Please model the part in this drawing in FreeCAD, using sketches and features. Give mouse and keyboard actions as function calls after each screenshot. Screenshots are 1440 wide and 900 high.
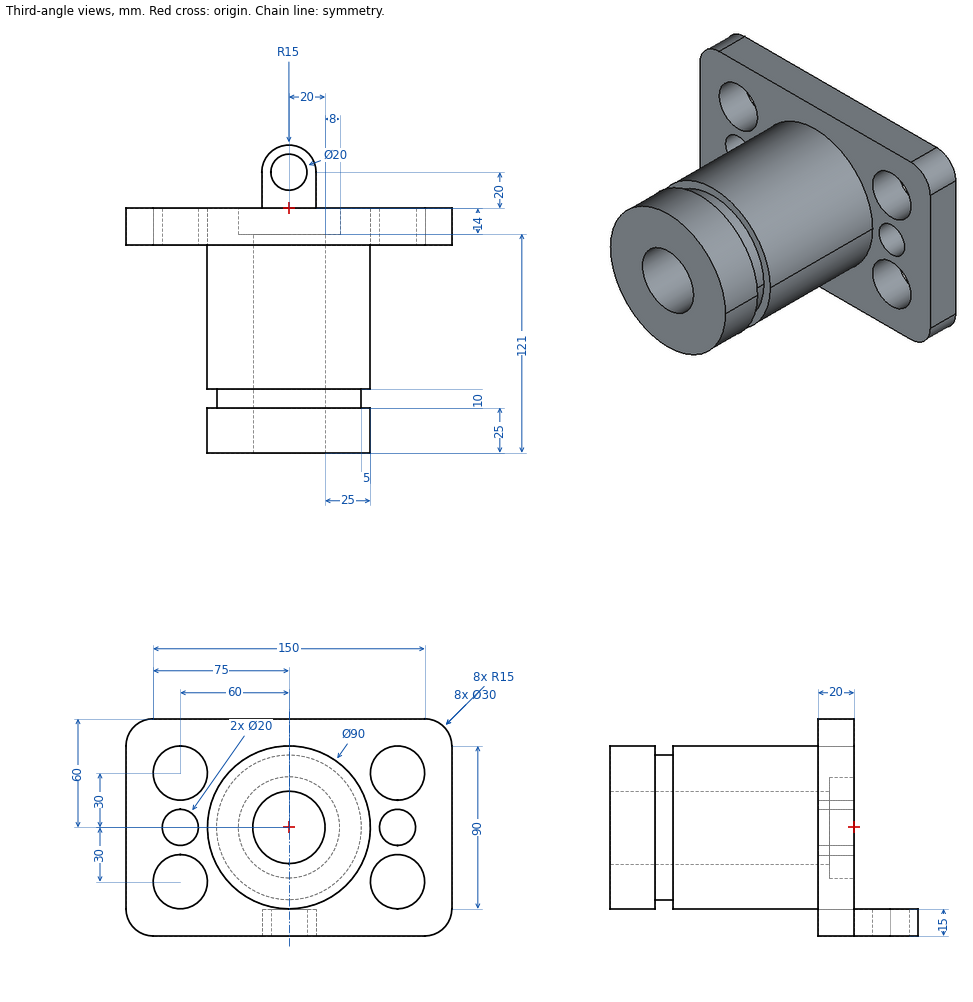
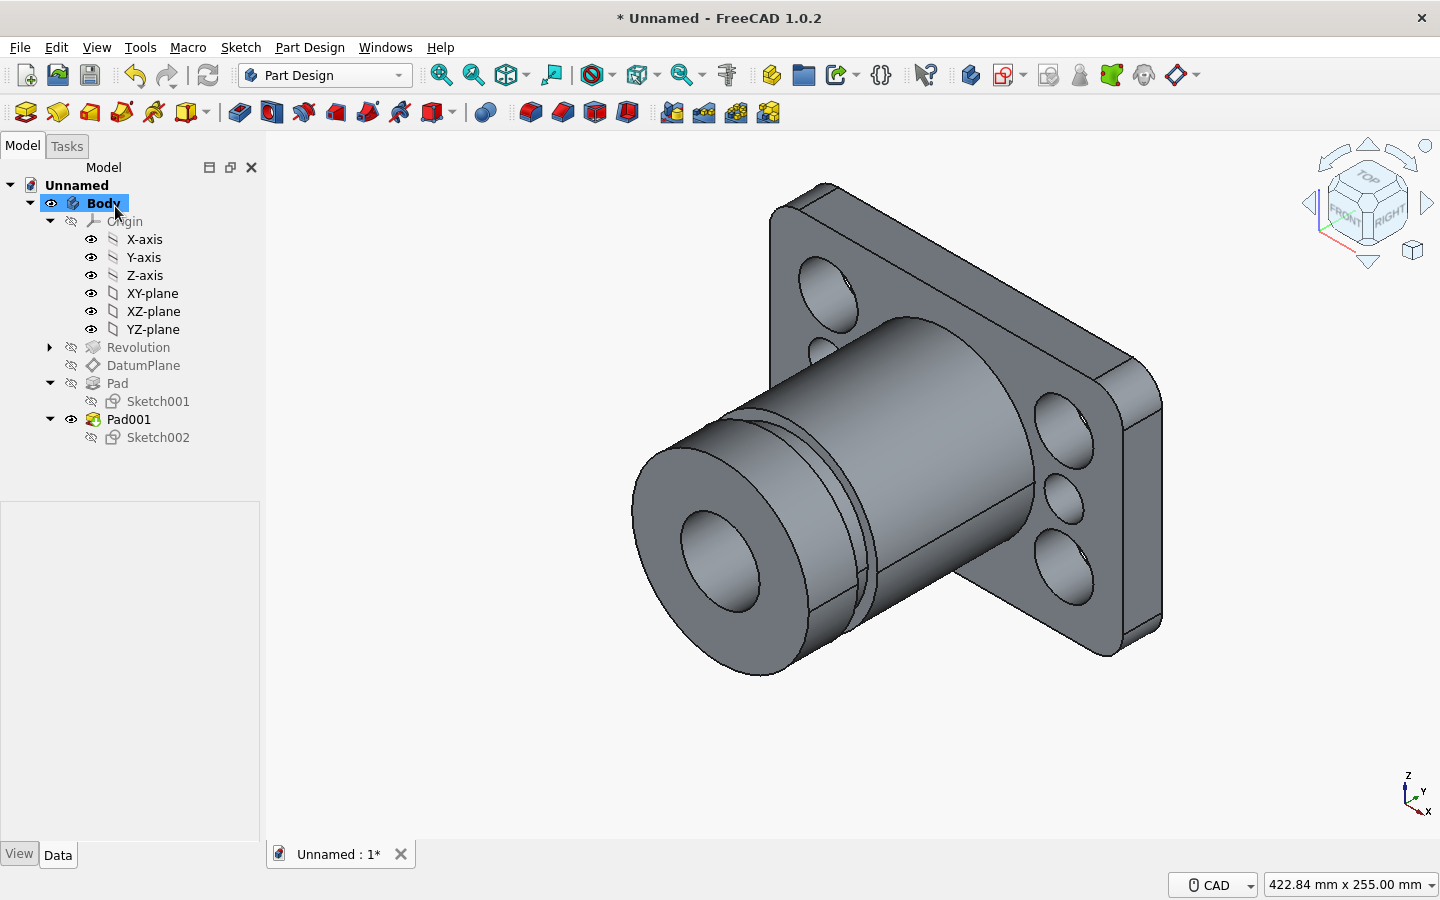
key(v)
key(f)